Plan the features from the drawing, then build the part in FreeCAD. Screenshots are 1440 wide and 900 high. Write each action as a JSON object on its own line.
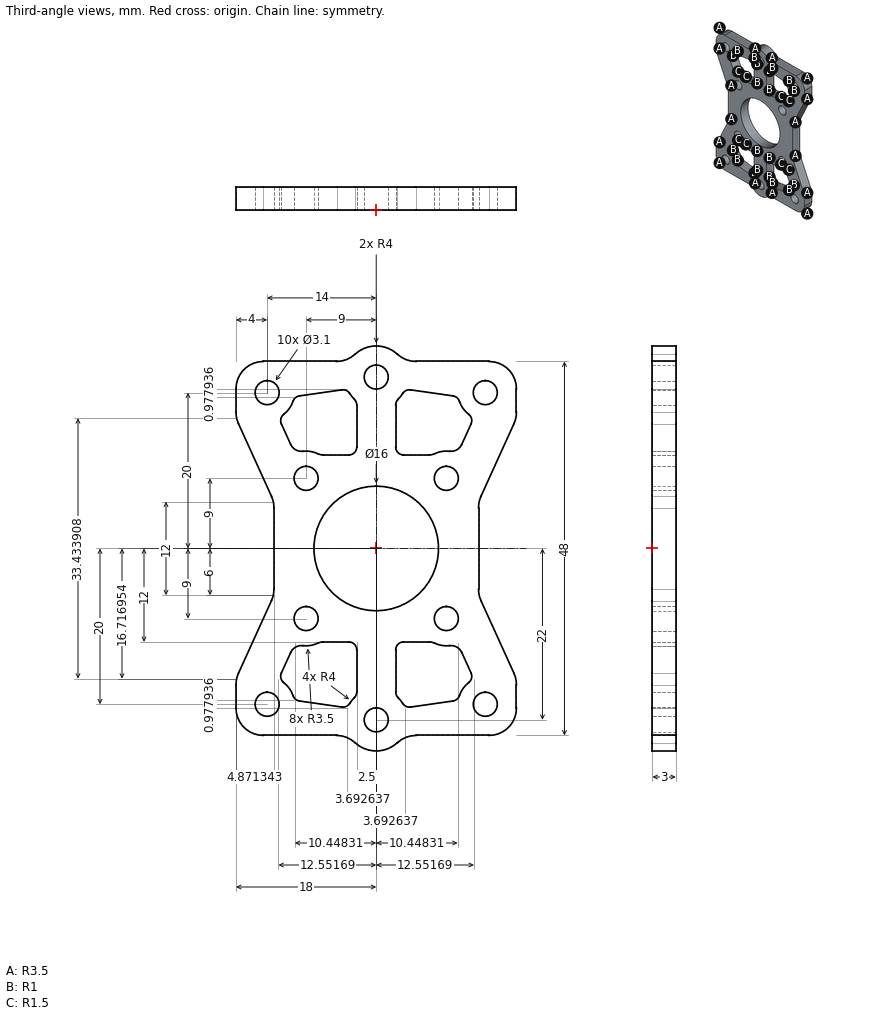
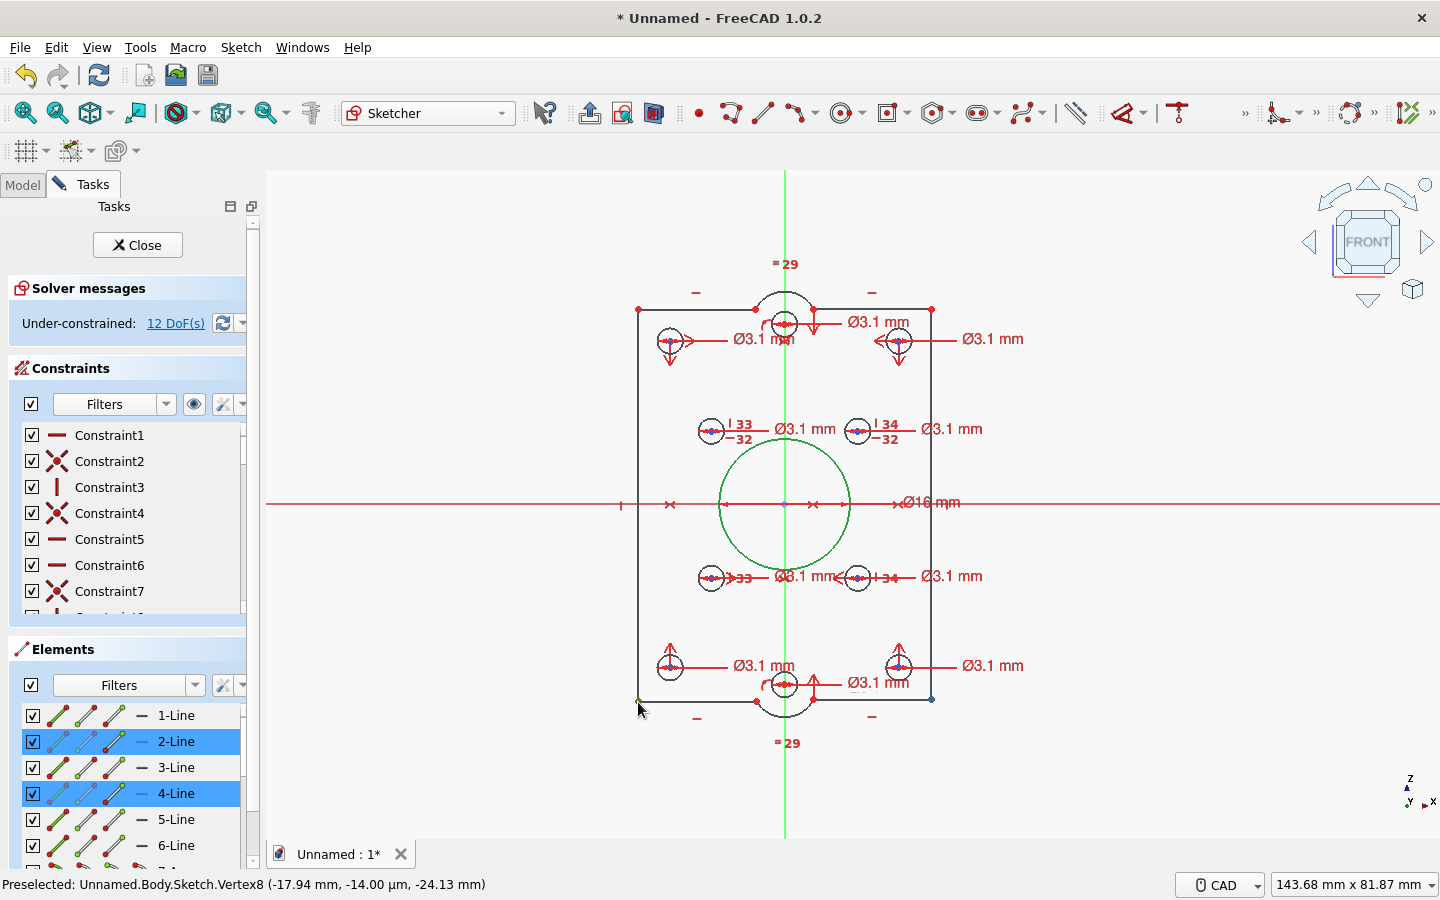
{"action": "left_click", "coordinate": [785, 767]}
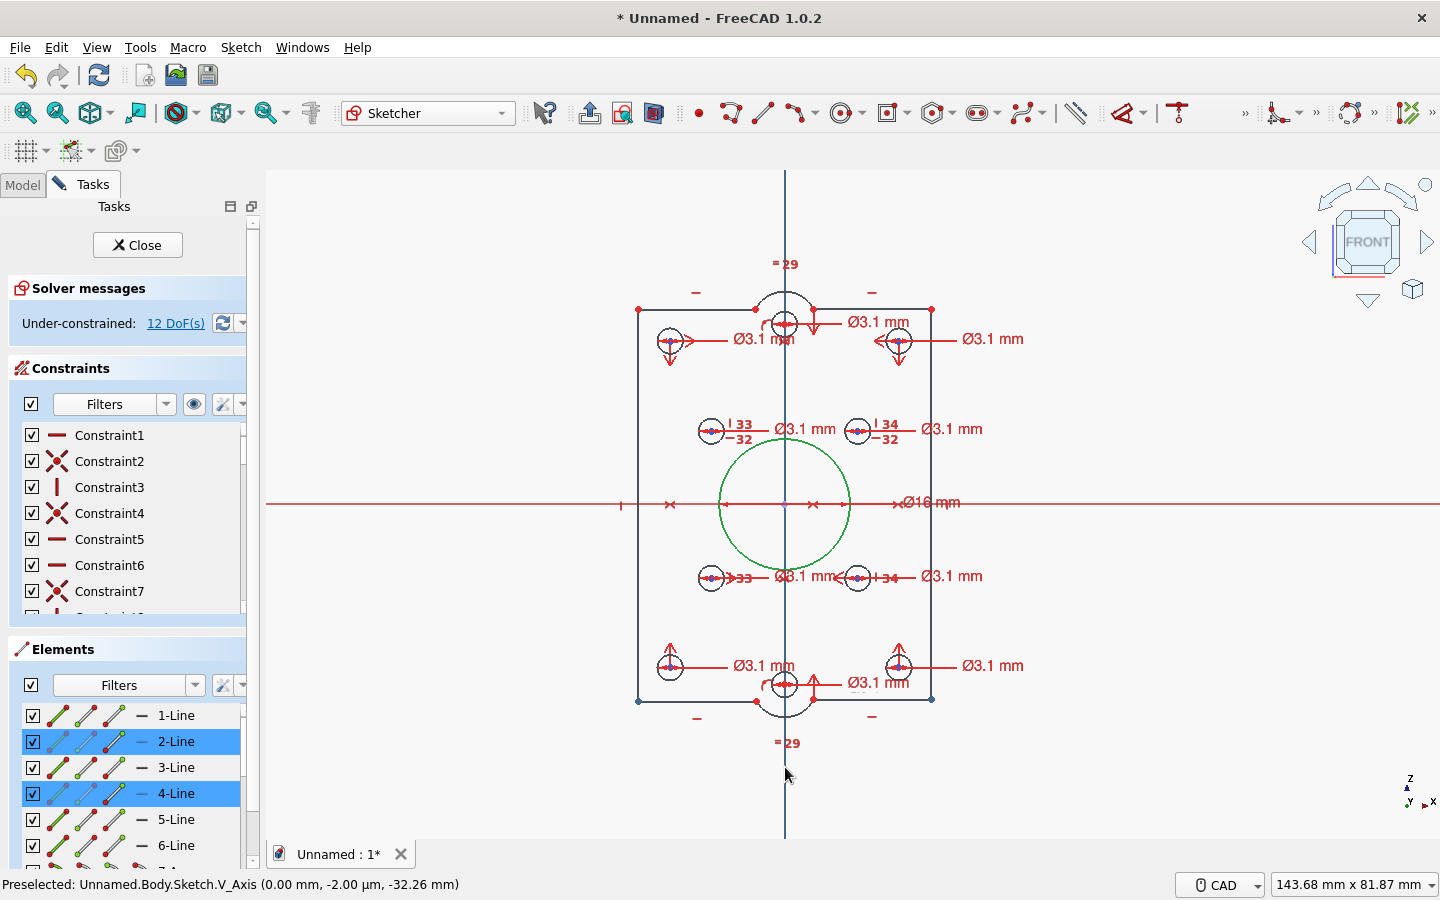
{"action": "key", "text": "s"}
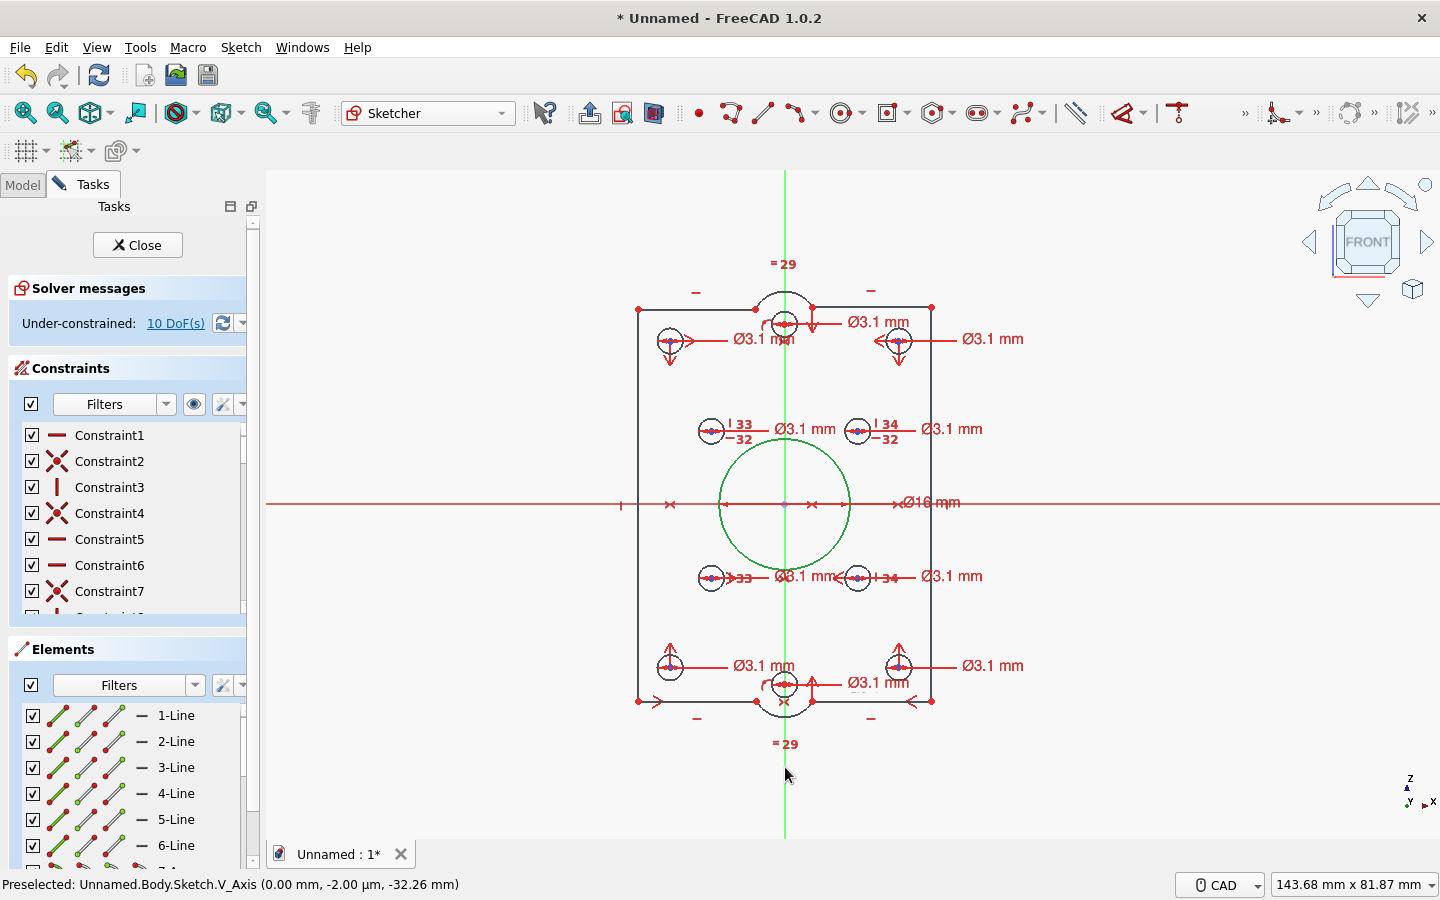
{"action": "left_click", "coordinate": [1122, 114]}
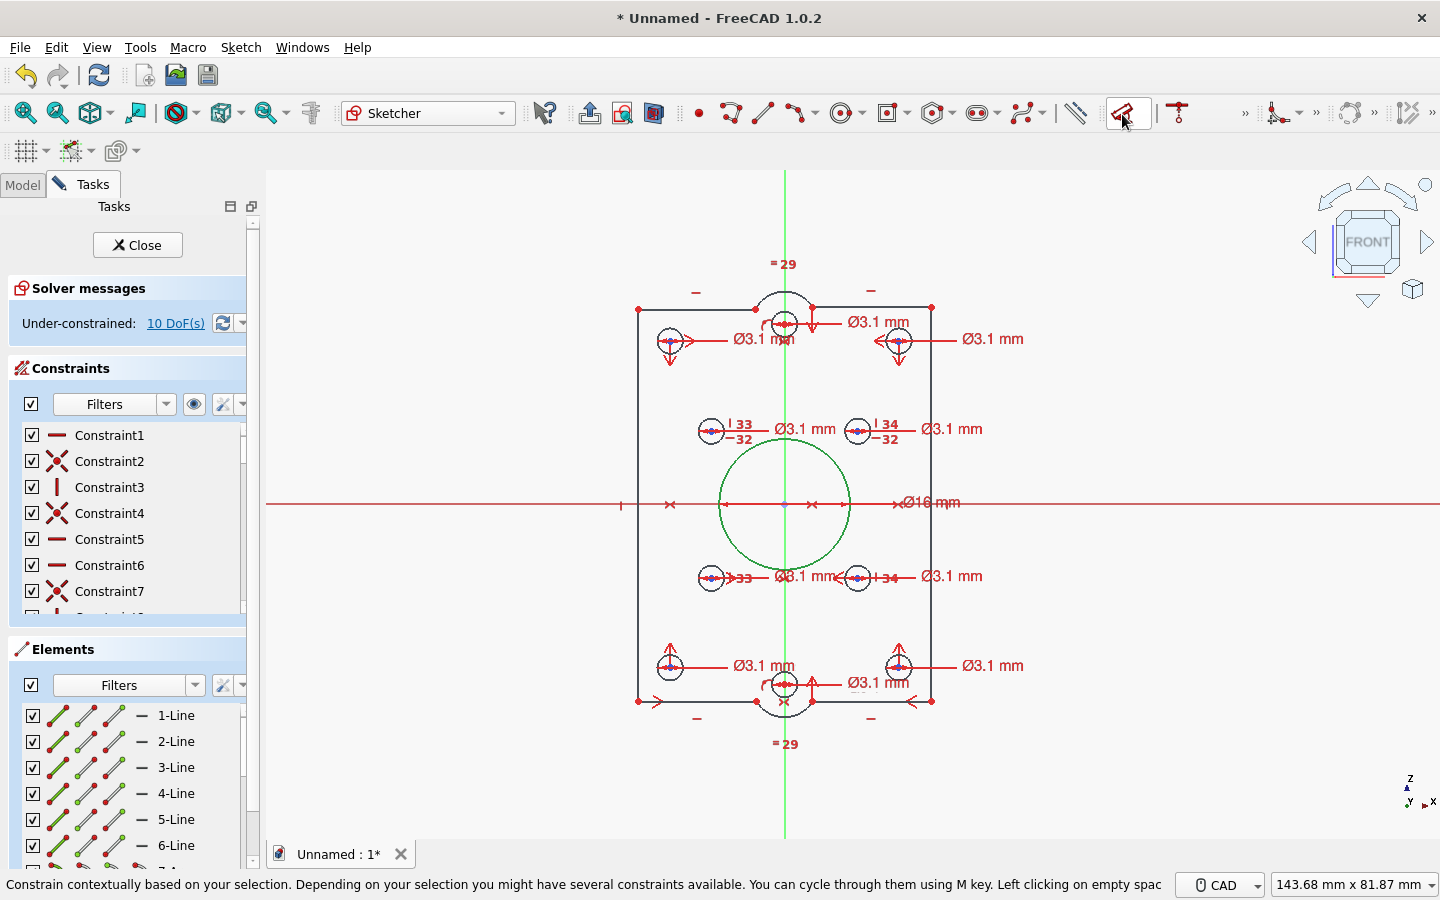
{"action": "left_click", "coordinate": [772, 715]}
{"action": "left_click", "coordinate": [760, 745]}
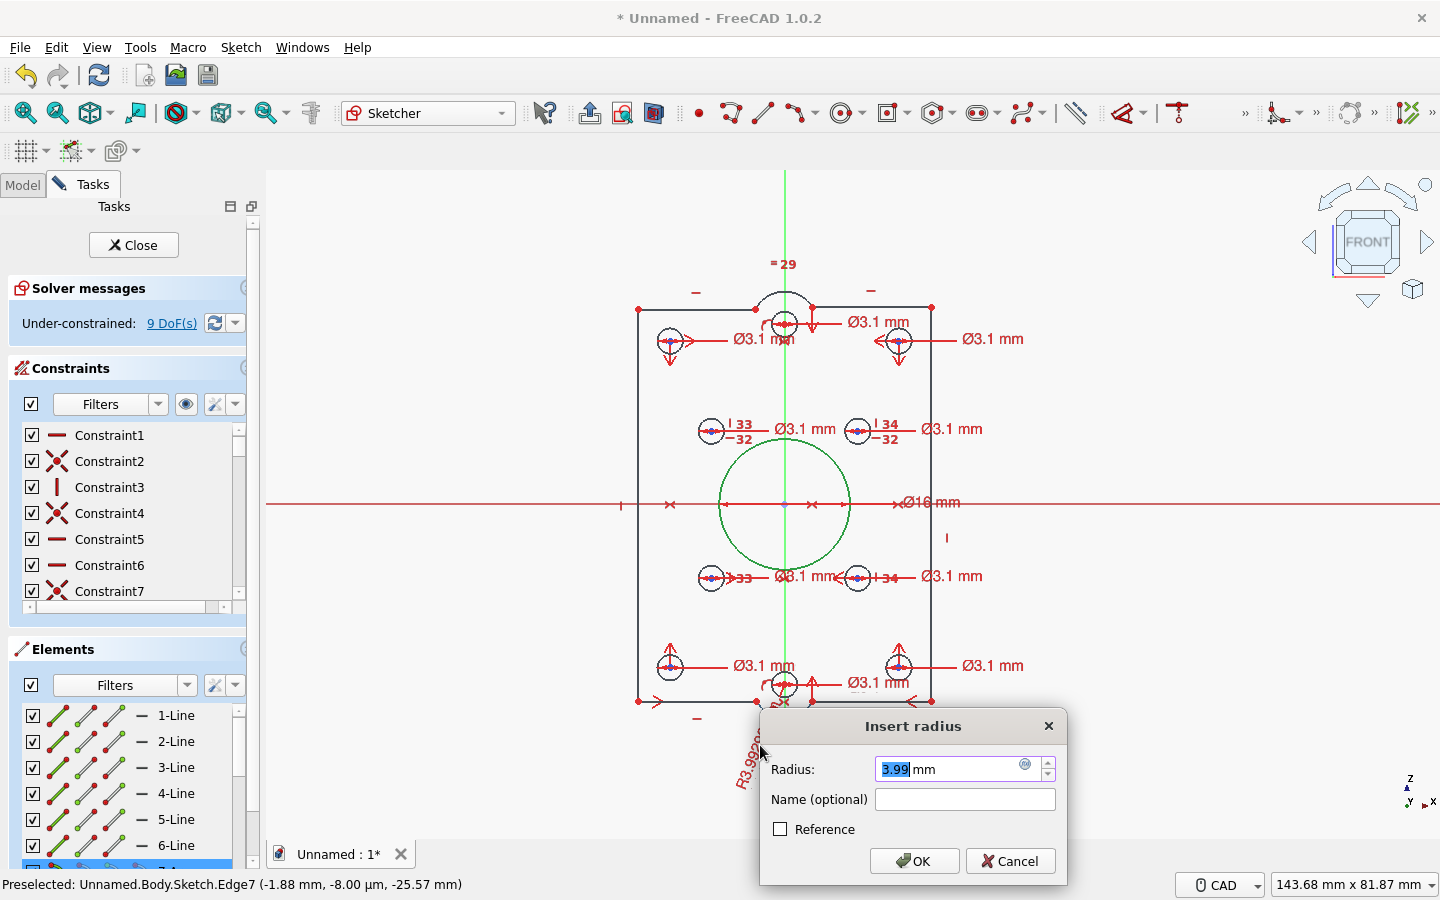
{"action": "type", "text": "4"}
{"action": "key", "text": "Return"}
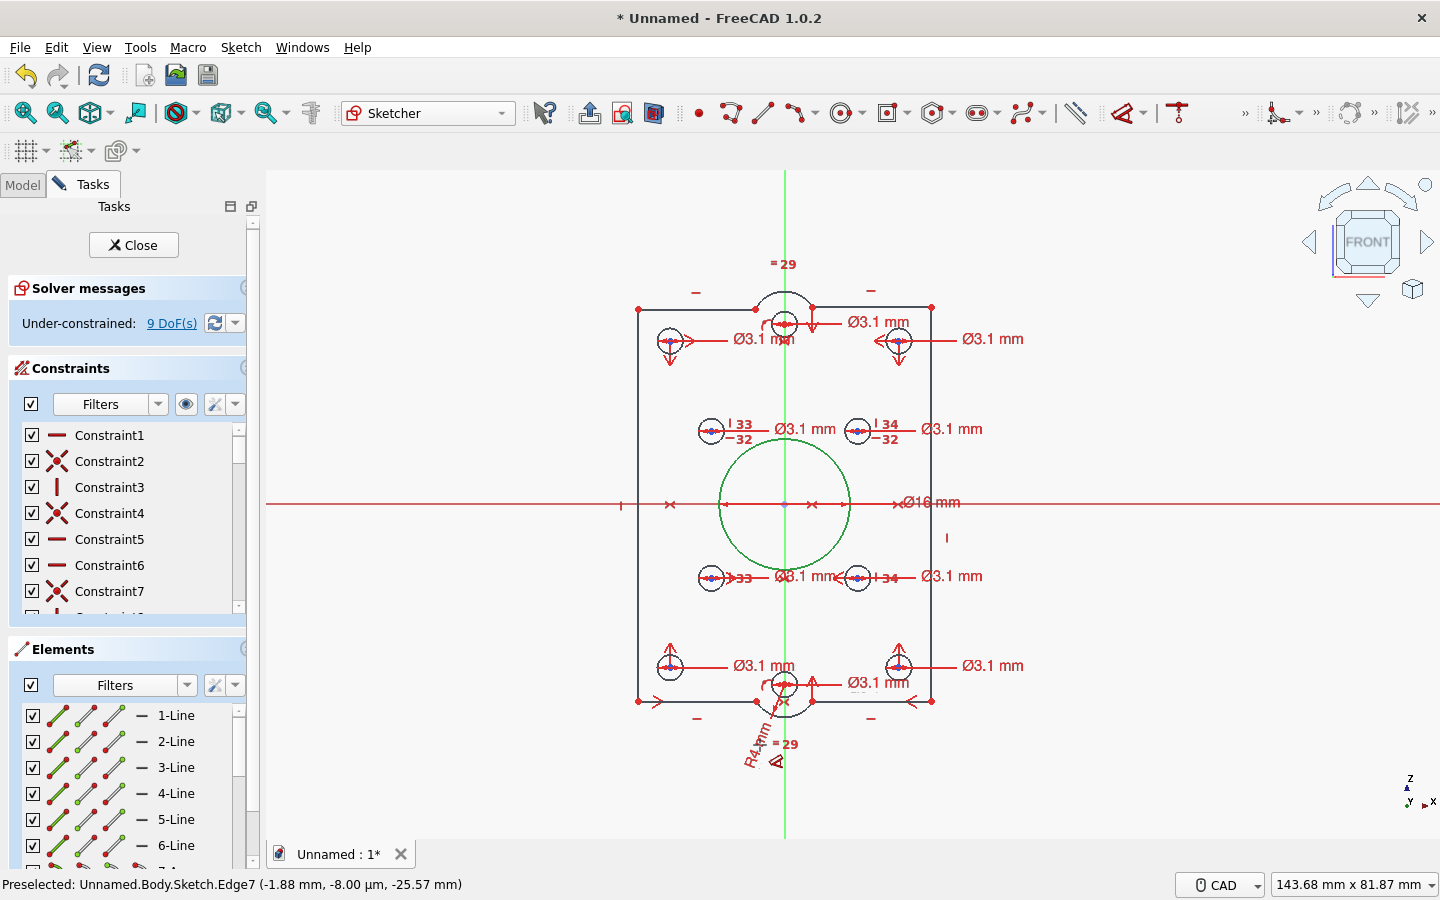
{"action": "left_click", "coordinate": [711, 431]}
{"action": "left_click", "coordinate": [748, 397]}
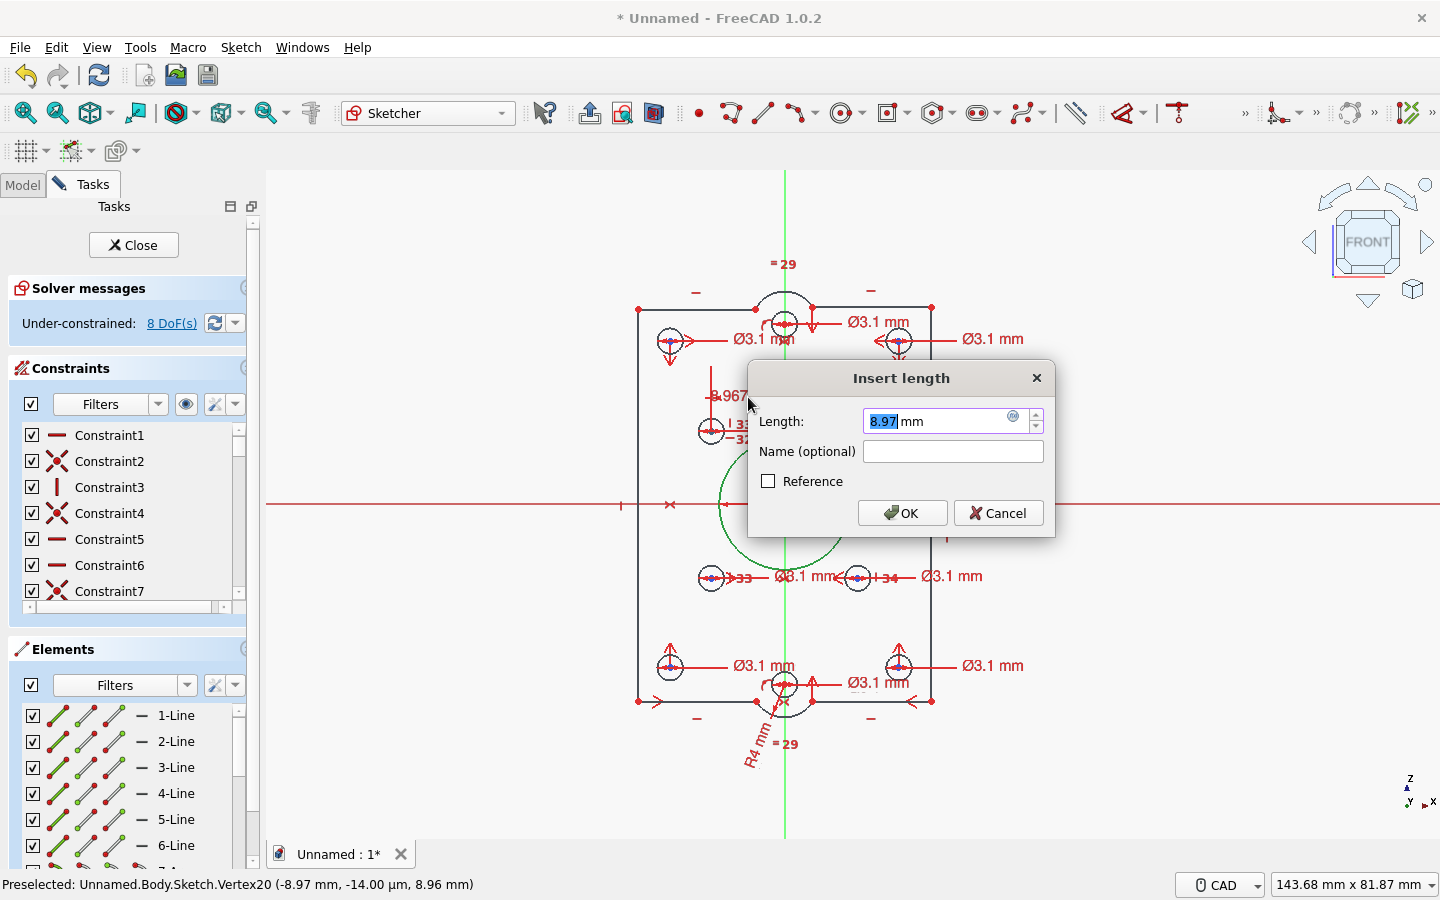
{"action": "type", "text": "9"}
{"action": "key", "text": "Return"}